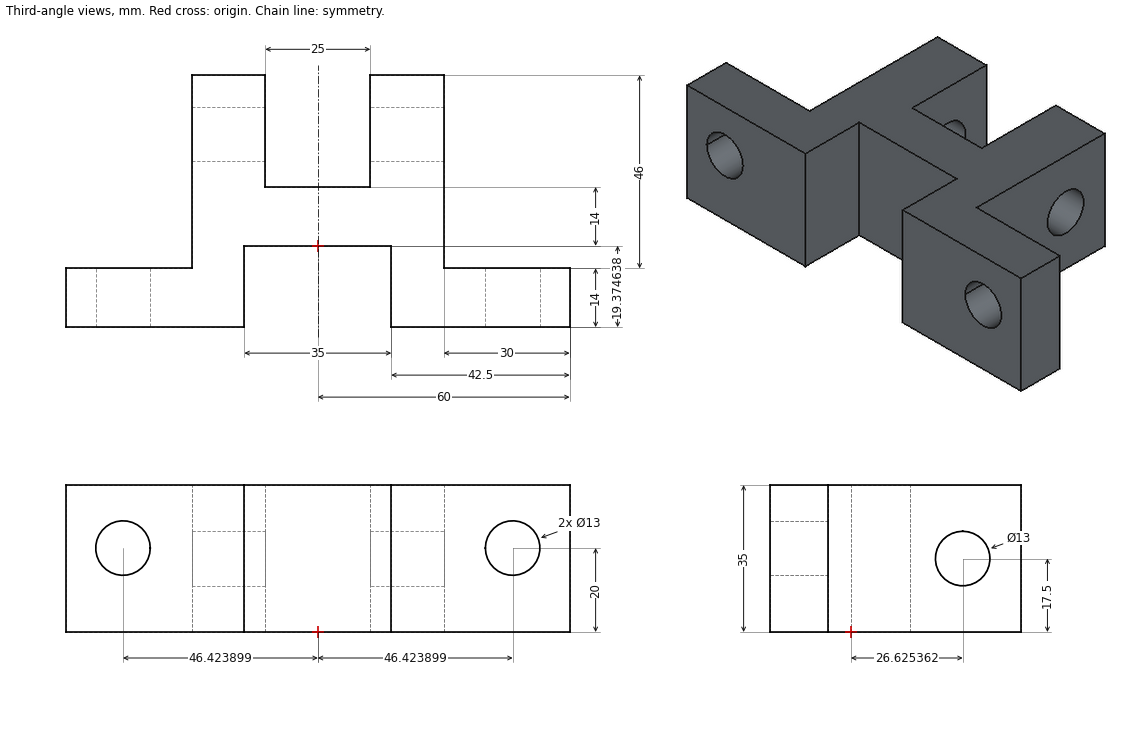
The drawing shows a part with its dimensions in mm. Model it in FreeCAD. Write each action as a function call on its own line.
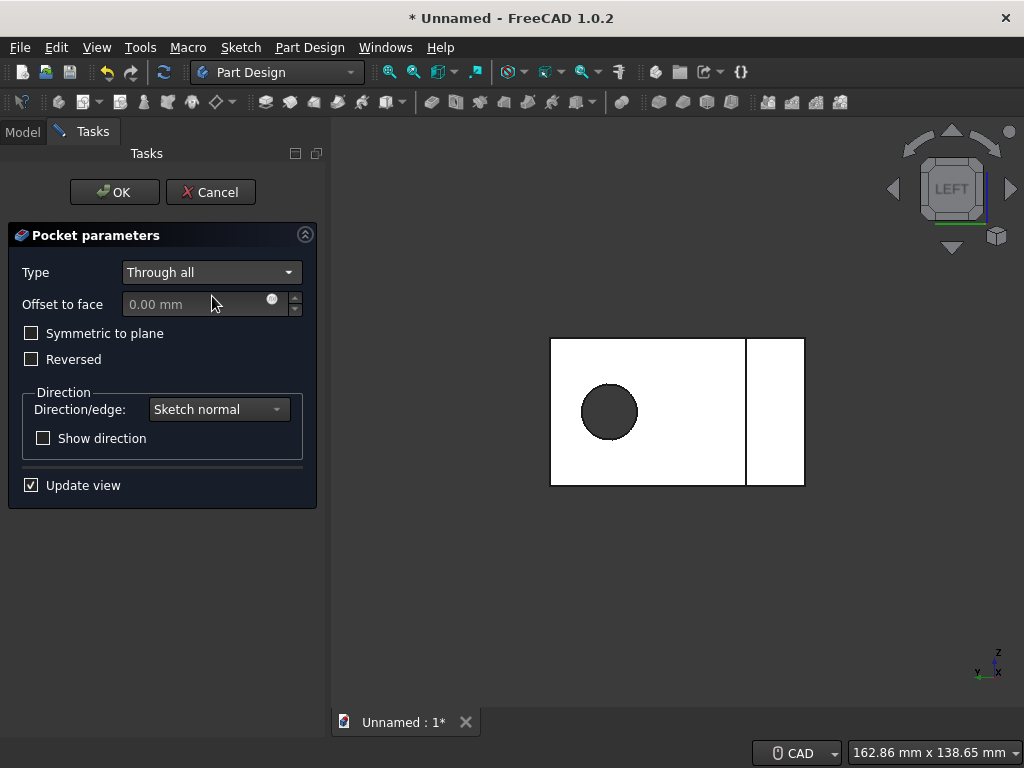
click(115, 192)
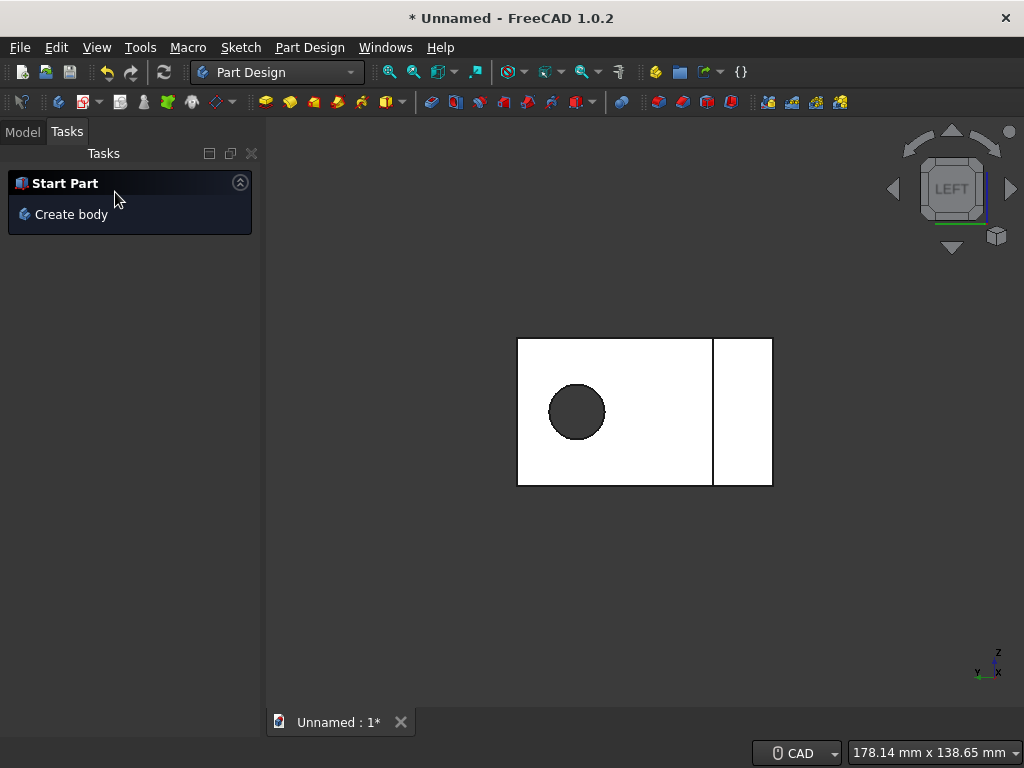
click(390, 72)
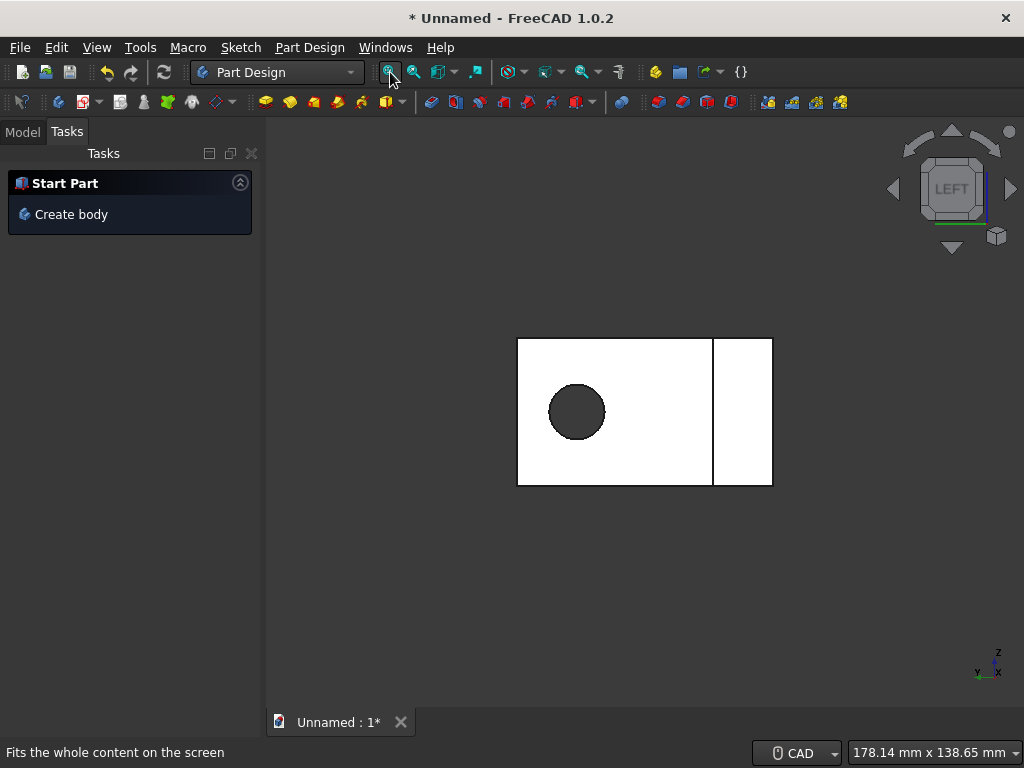
key(4)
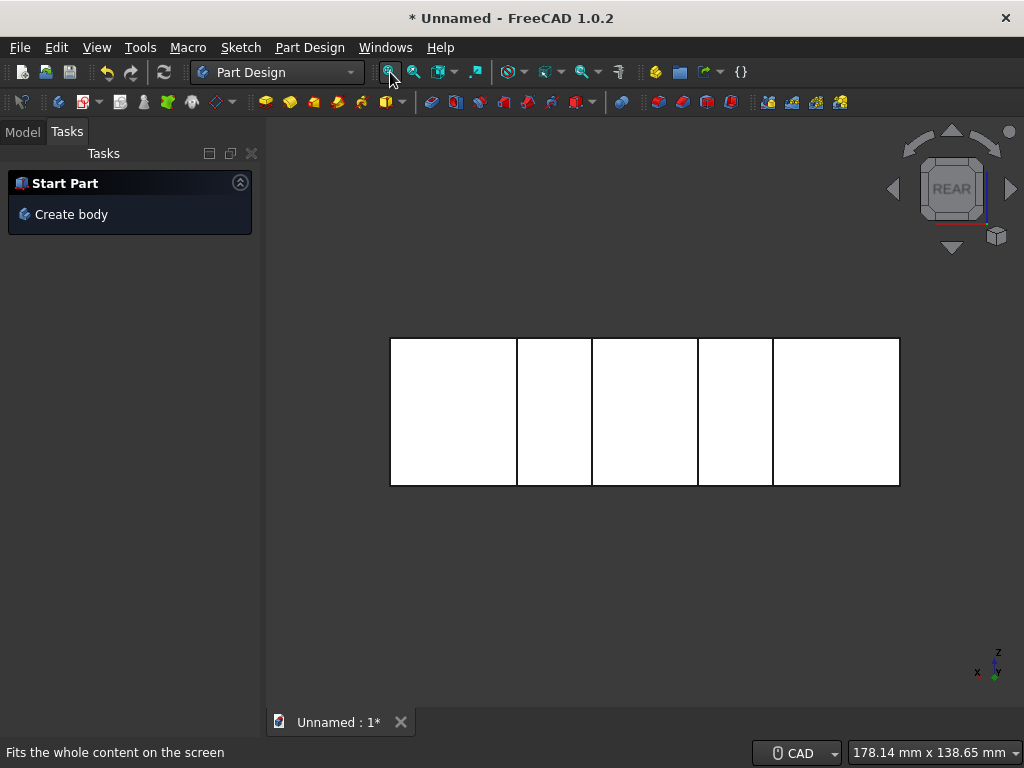
click(454, 411)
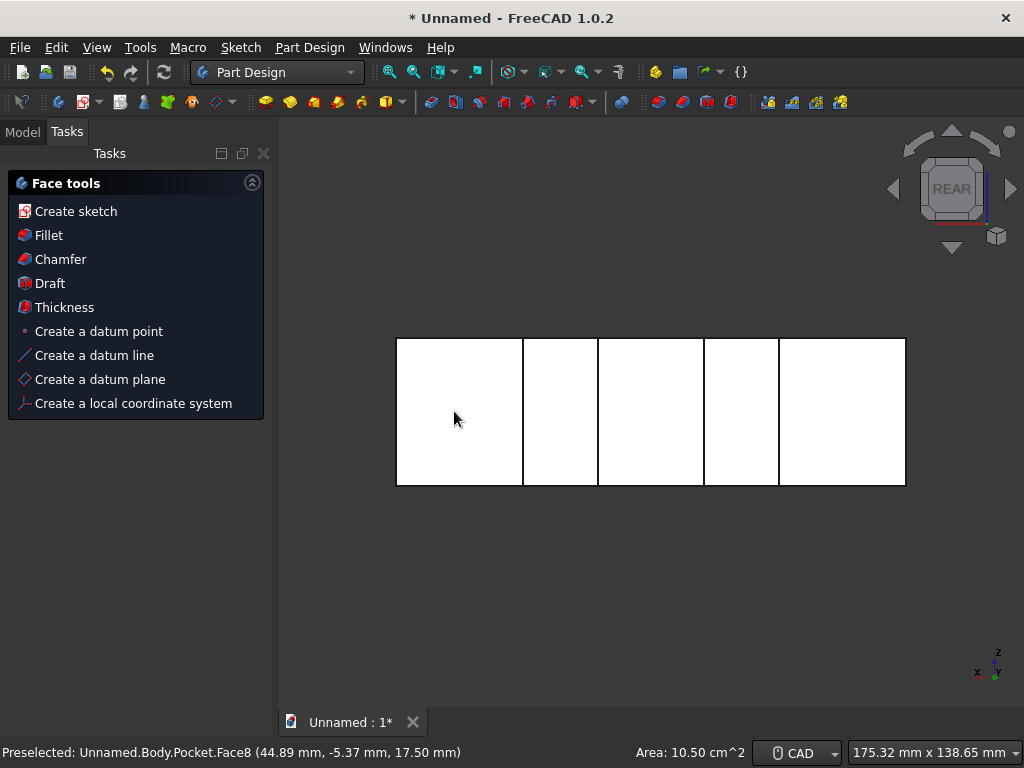
click(84, 102)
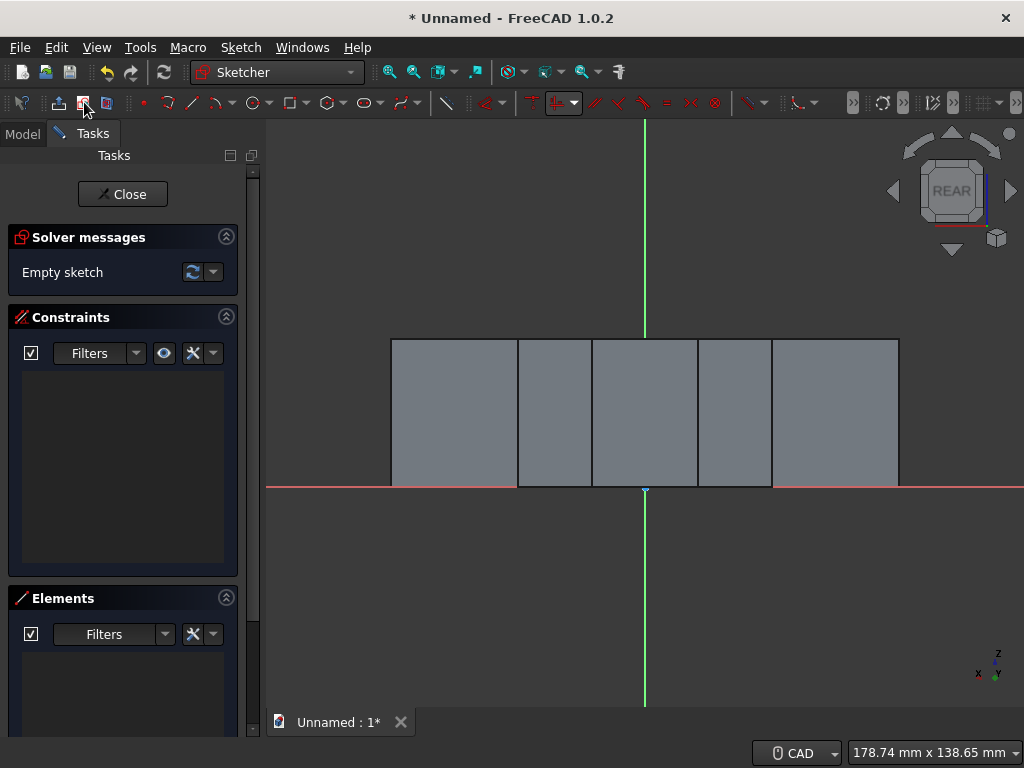
scroll(294, 332, down, 1)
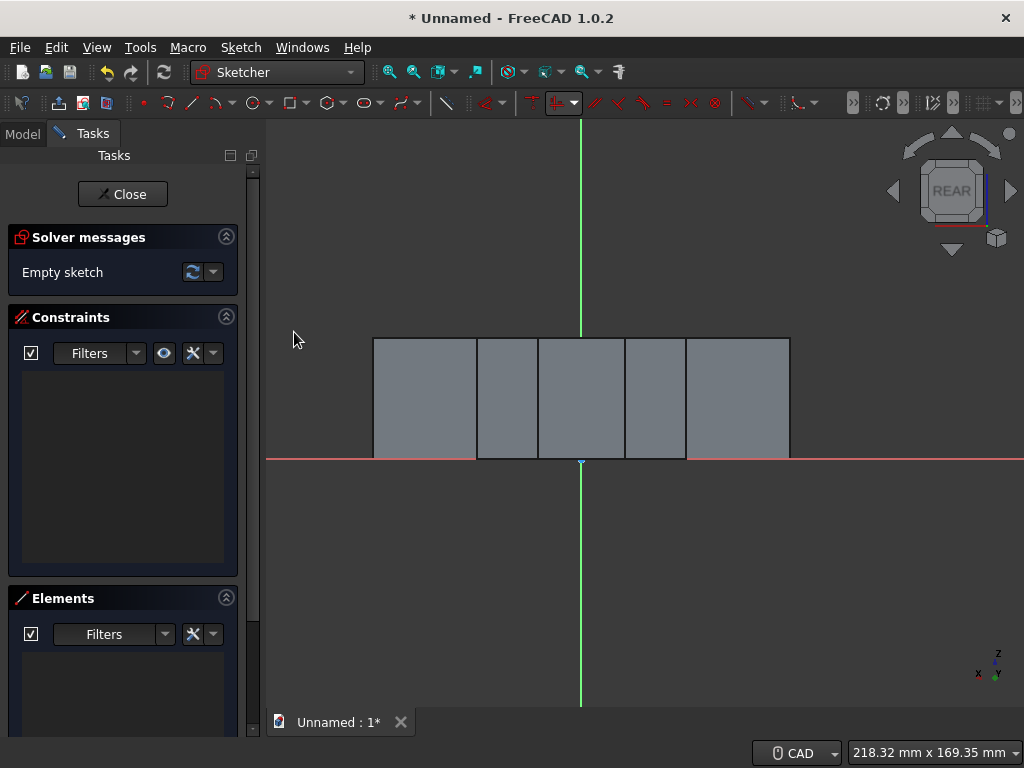
click(254, 104)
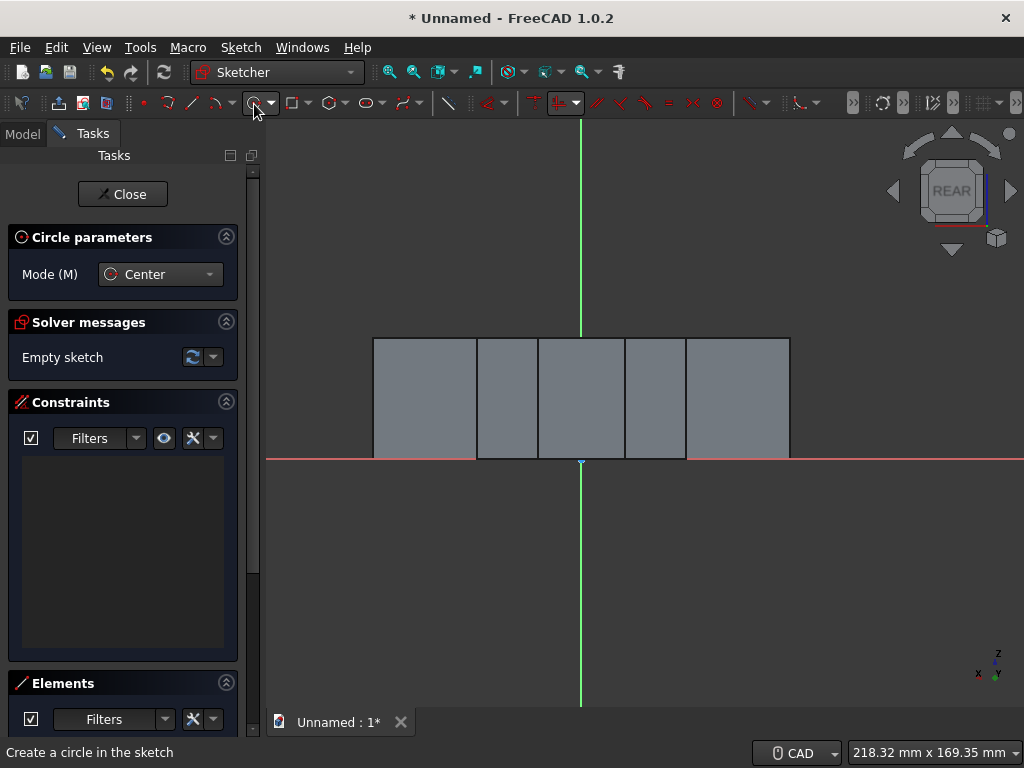
click(420, 390)
click(436, 374)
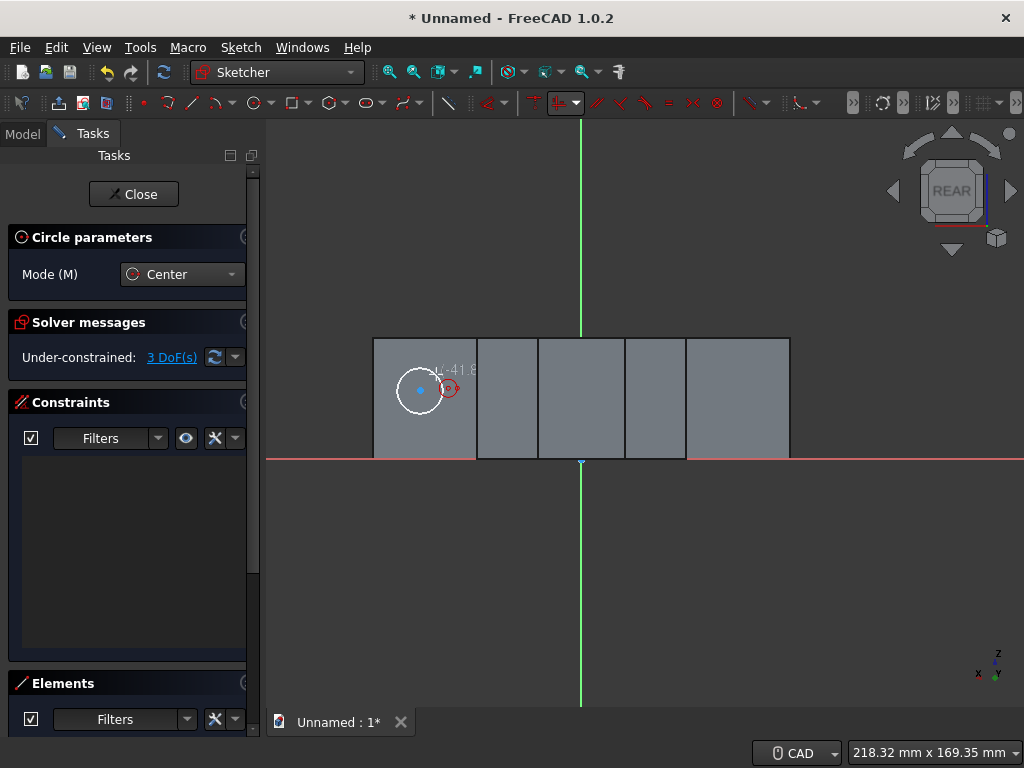
click(743, 390)
click(759, 374)
key(Escape)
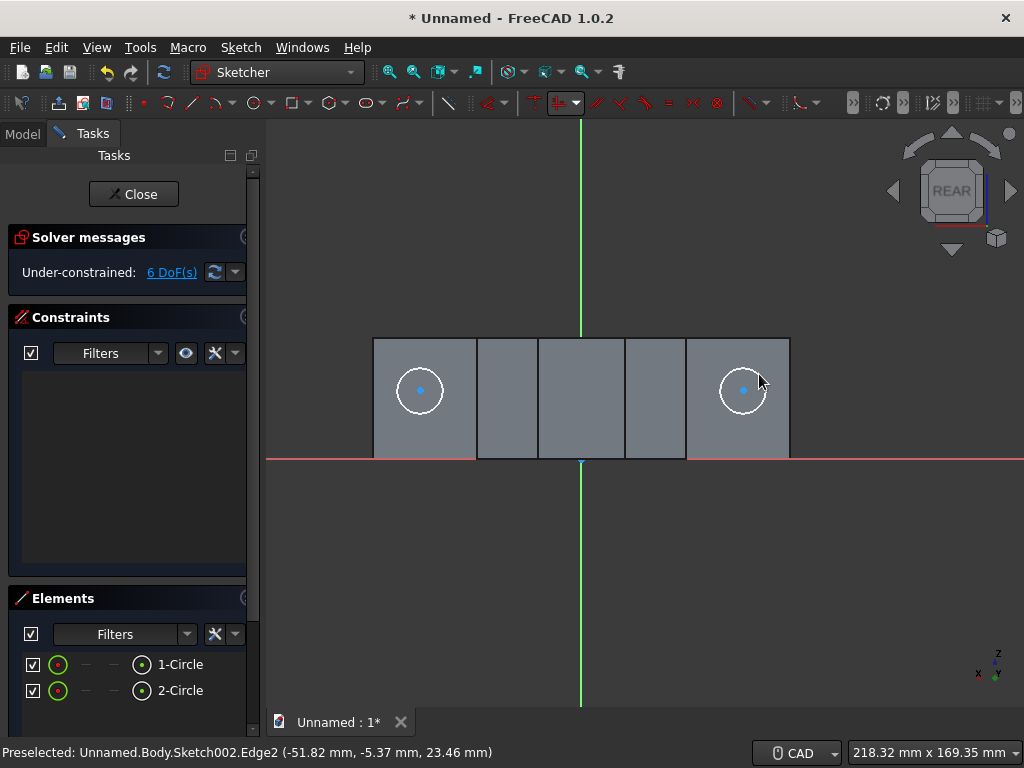
click(436, 375)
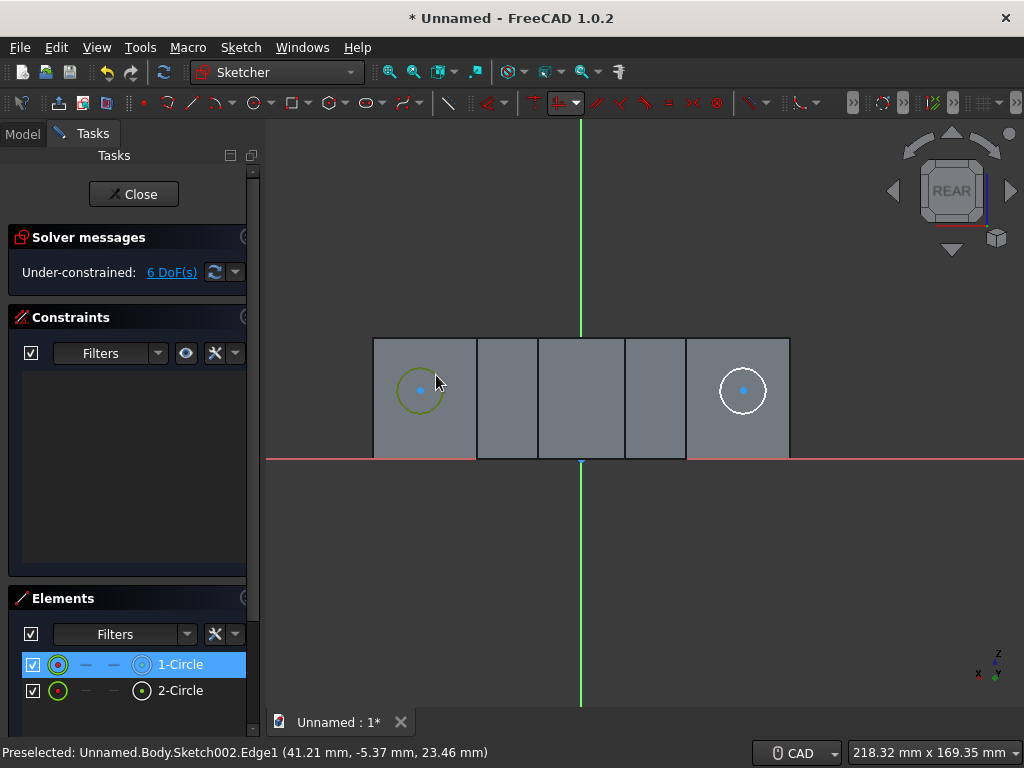
click(759, 375)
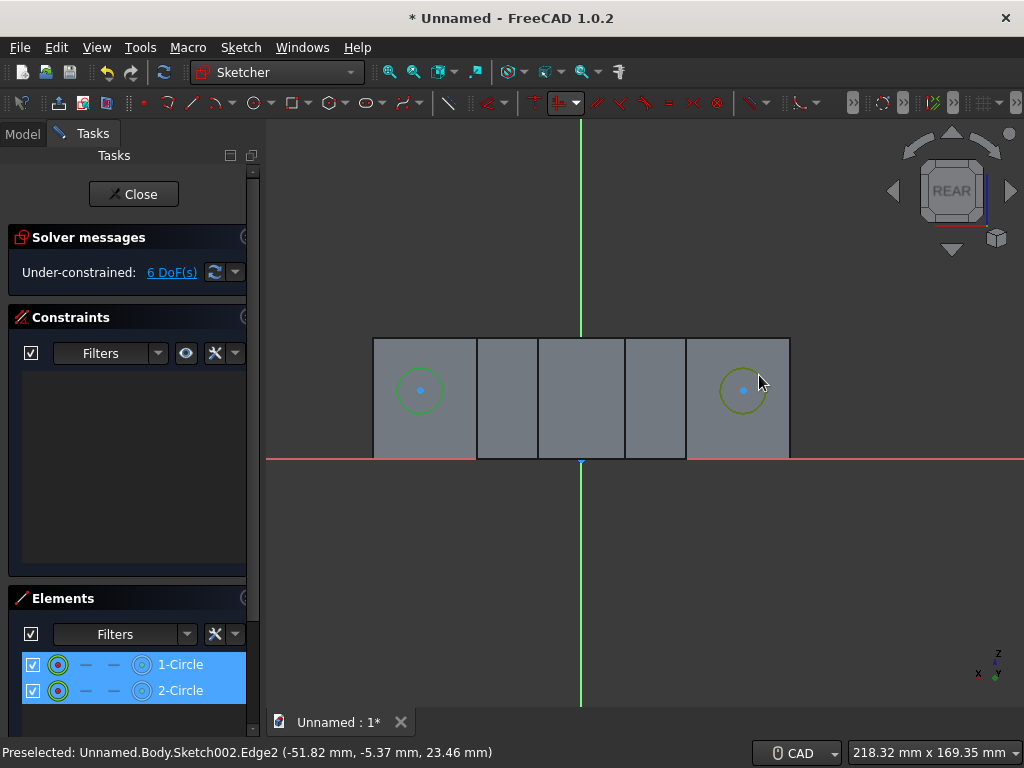
click(670, 104)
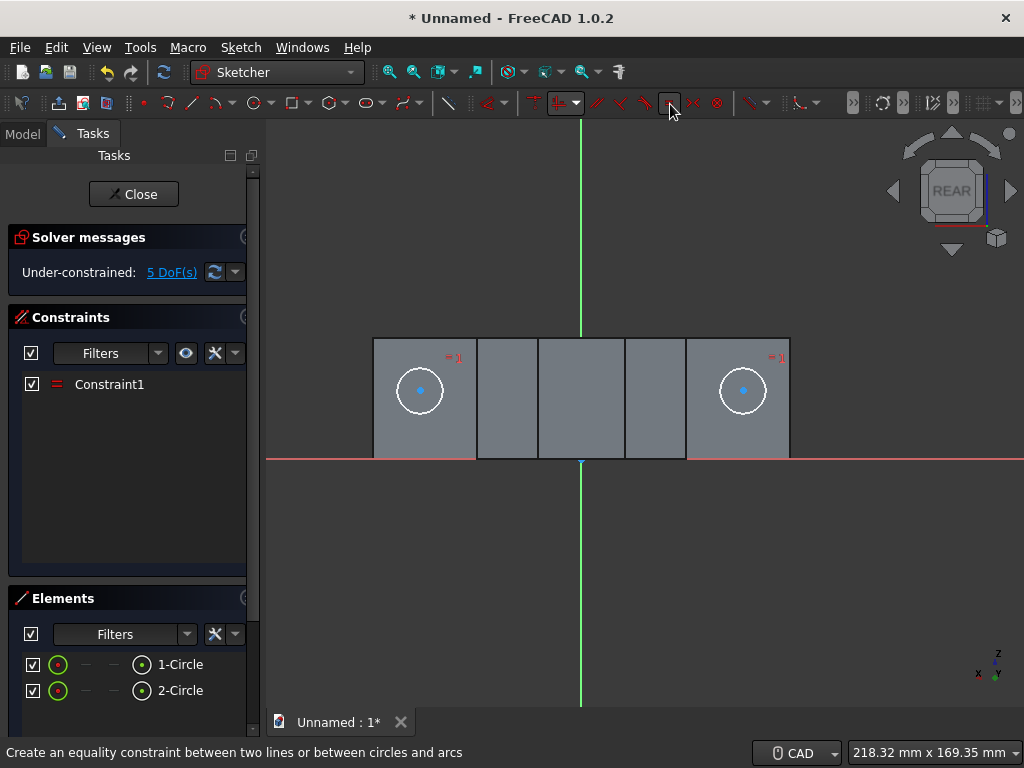
click(420, 391)